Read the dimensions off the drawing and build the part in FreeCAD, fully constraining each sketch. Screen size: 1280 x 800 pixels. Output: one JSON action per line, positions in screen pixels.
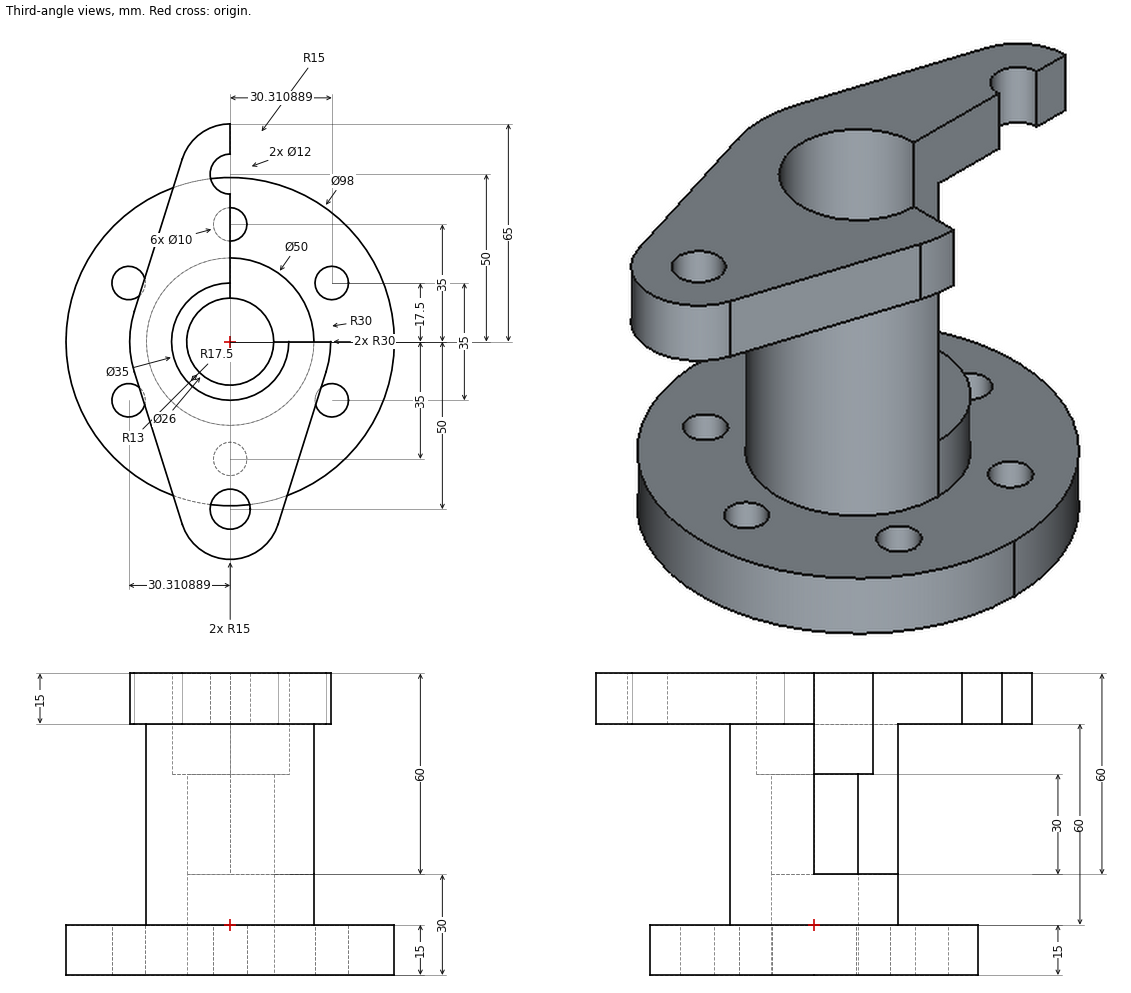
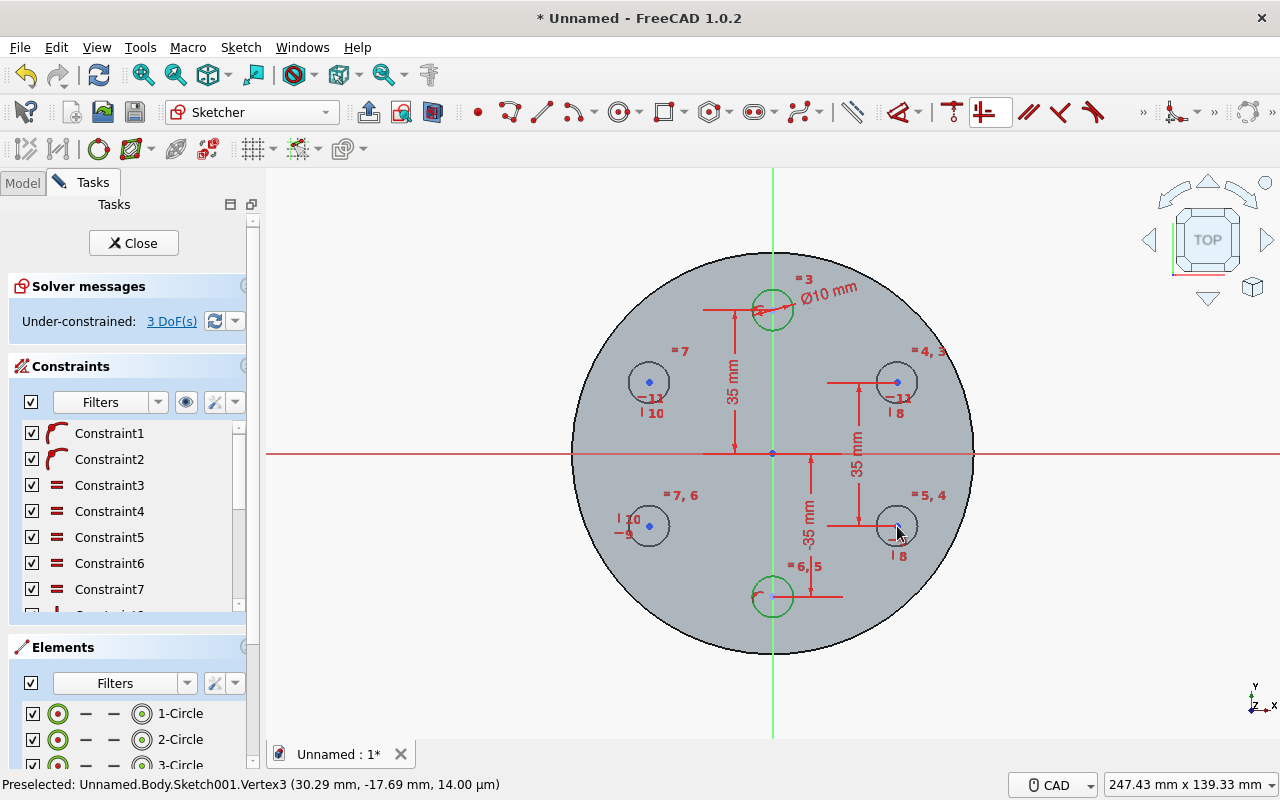
{"action": "left_click", "coordinate": [897, 383]}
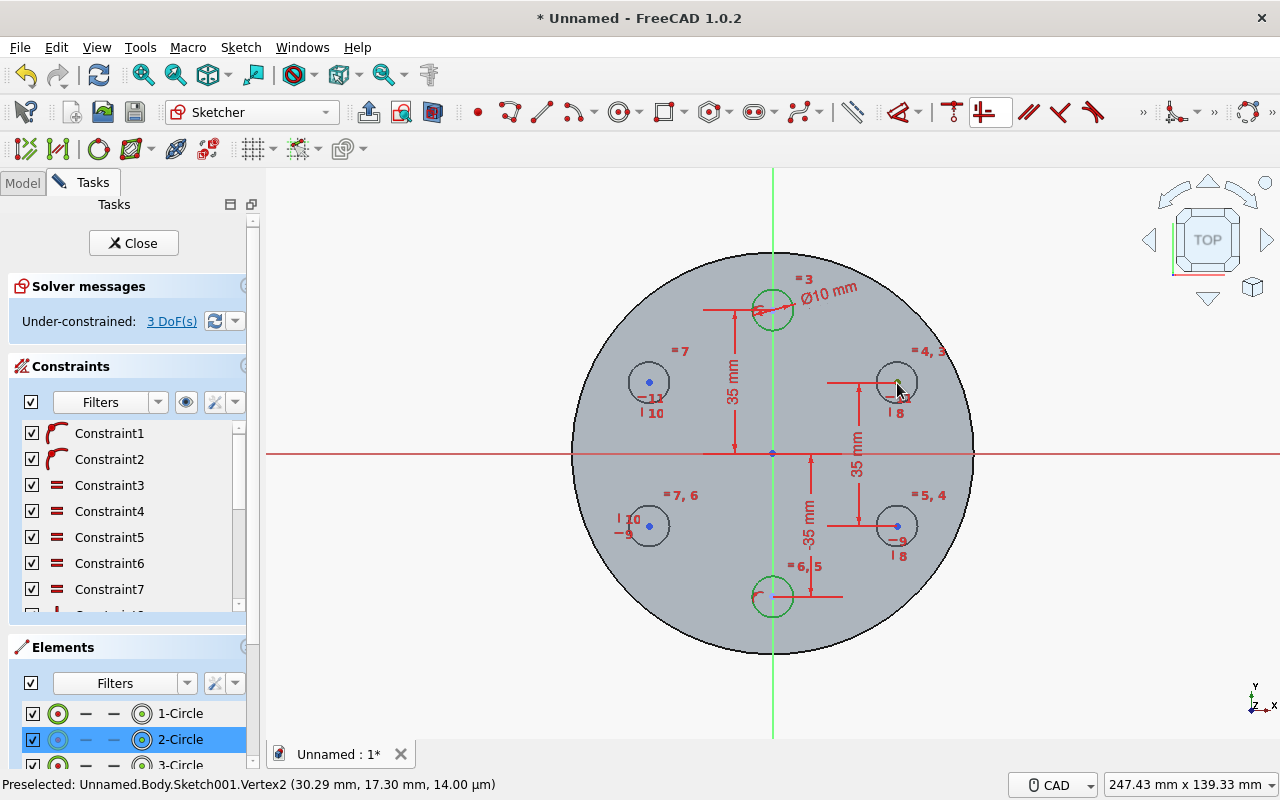
{"action": "key", "text": "i"}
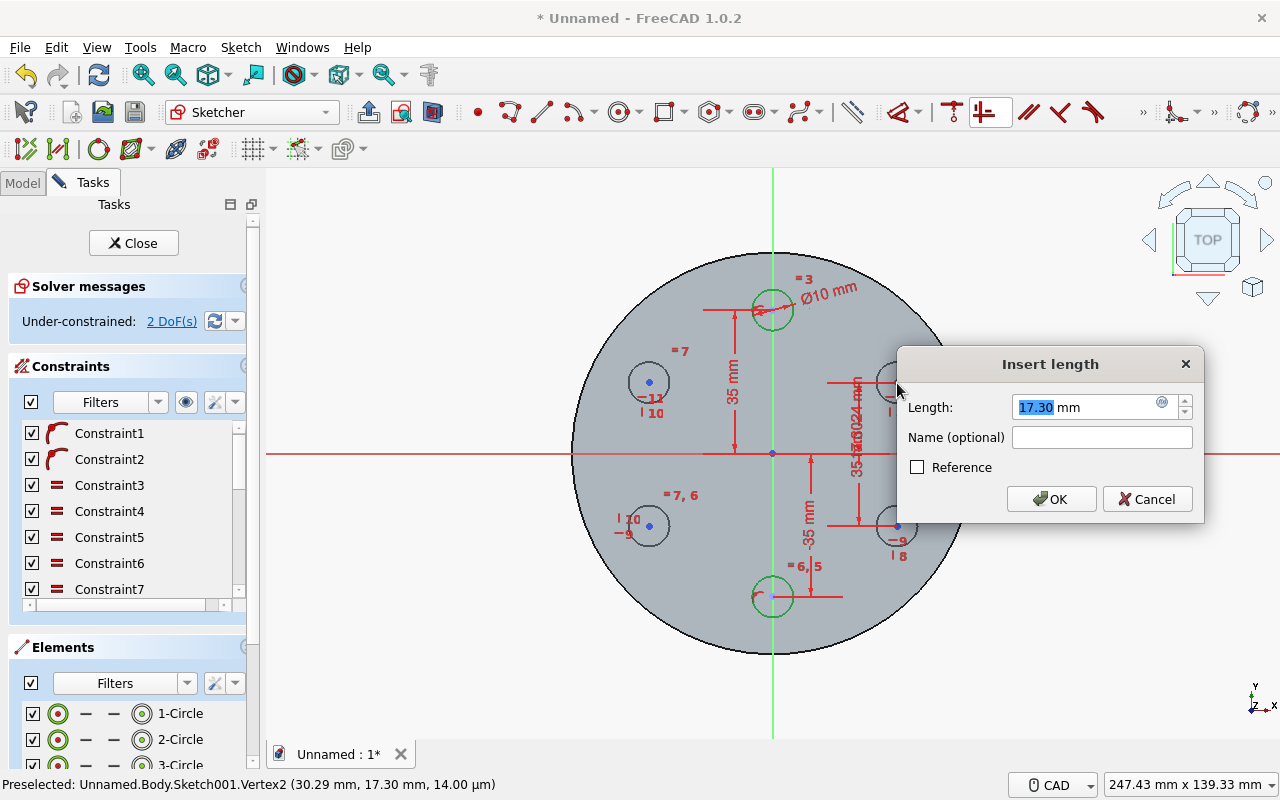
{"action": "type", "text": "17.5"}
{"action": "key", "text": "Return"}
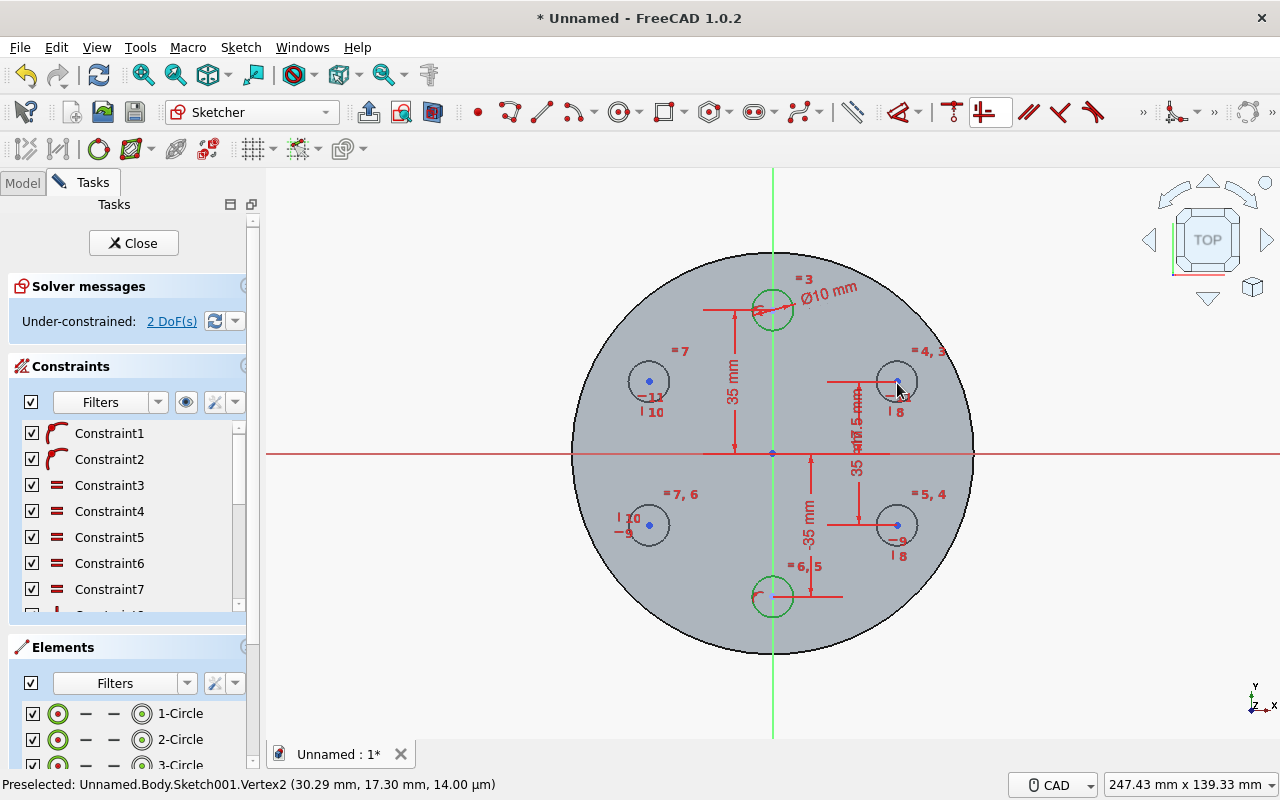
{"action": "left_click", "coordinate": [897, 382]}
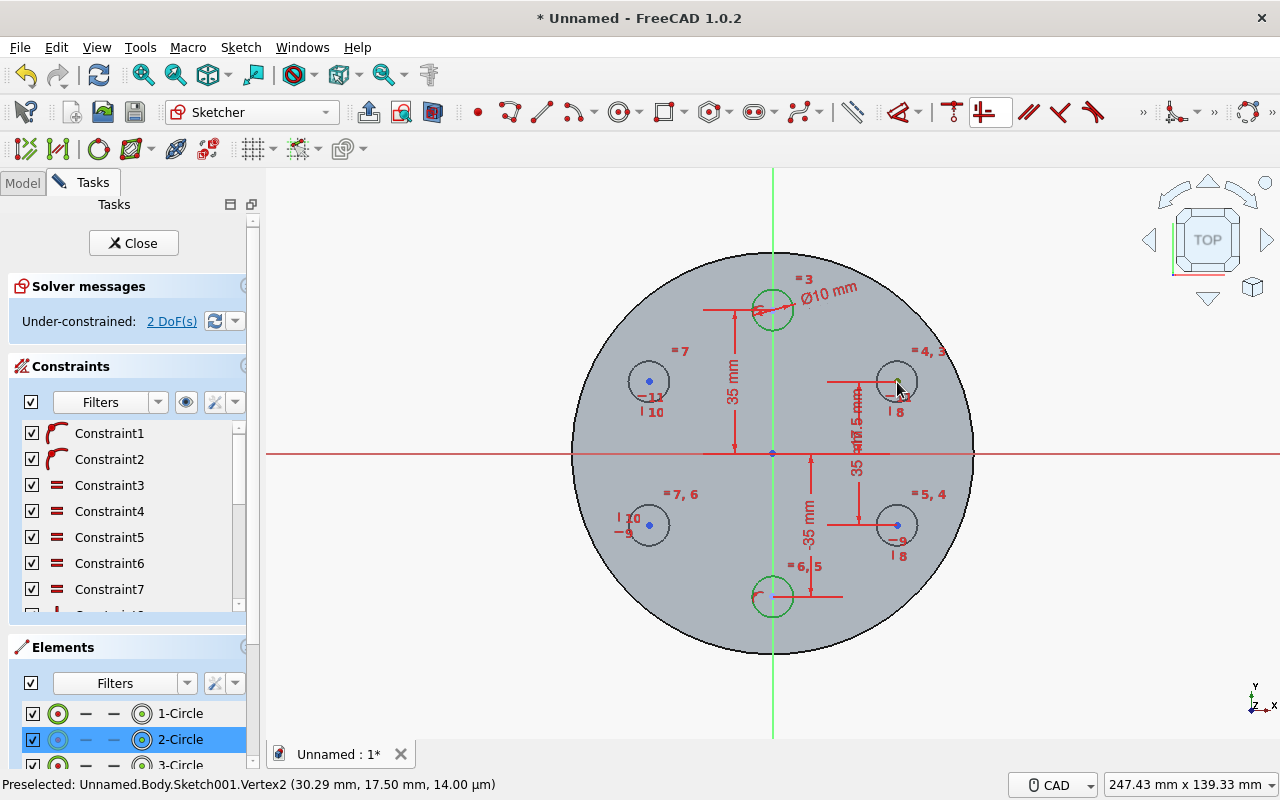
{"action": "key", "text": "l"}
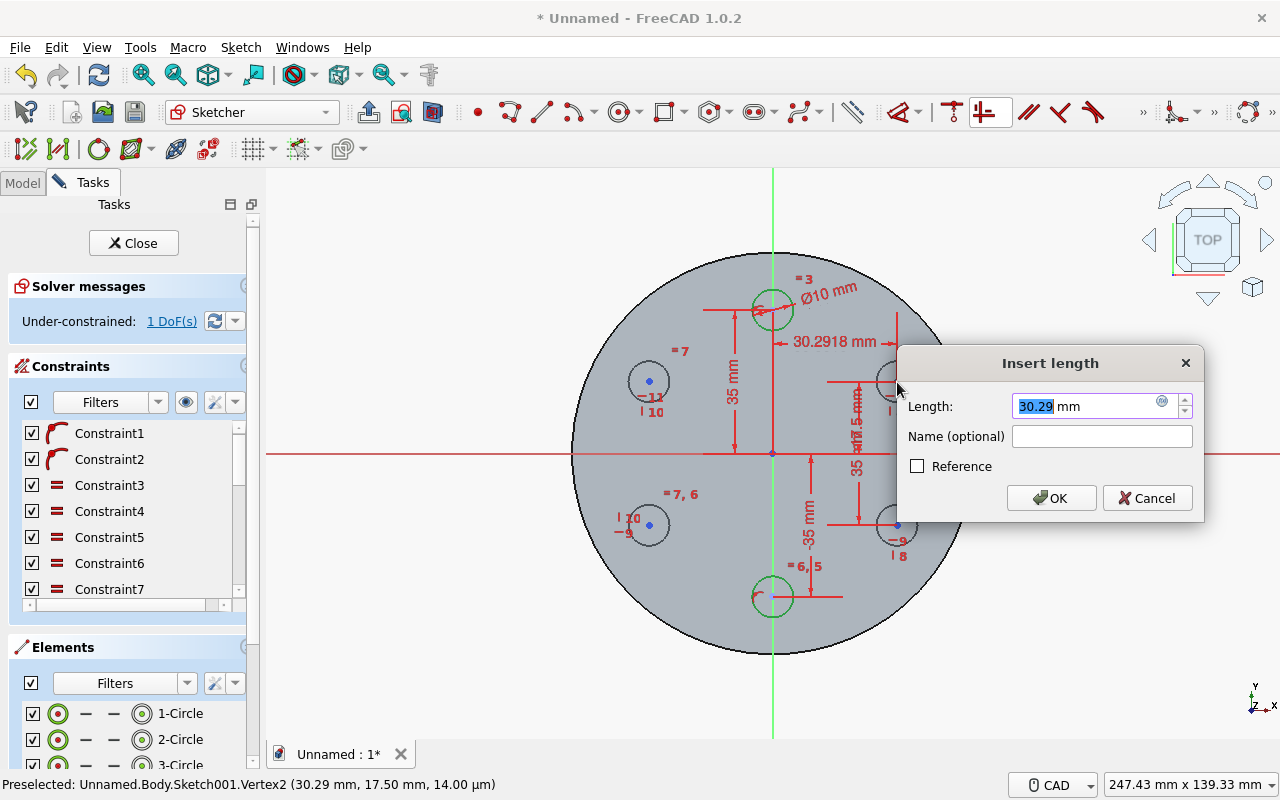
{"action": "type", "text": "30.310889"}
{"action": "key", "text": "Return"}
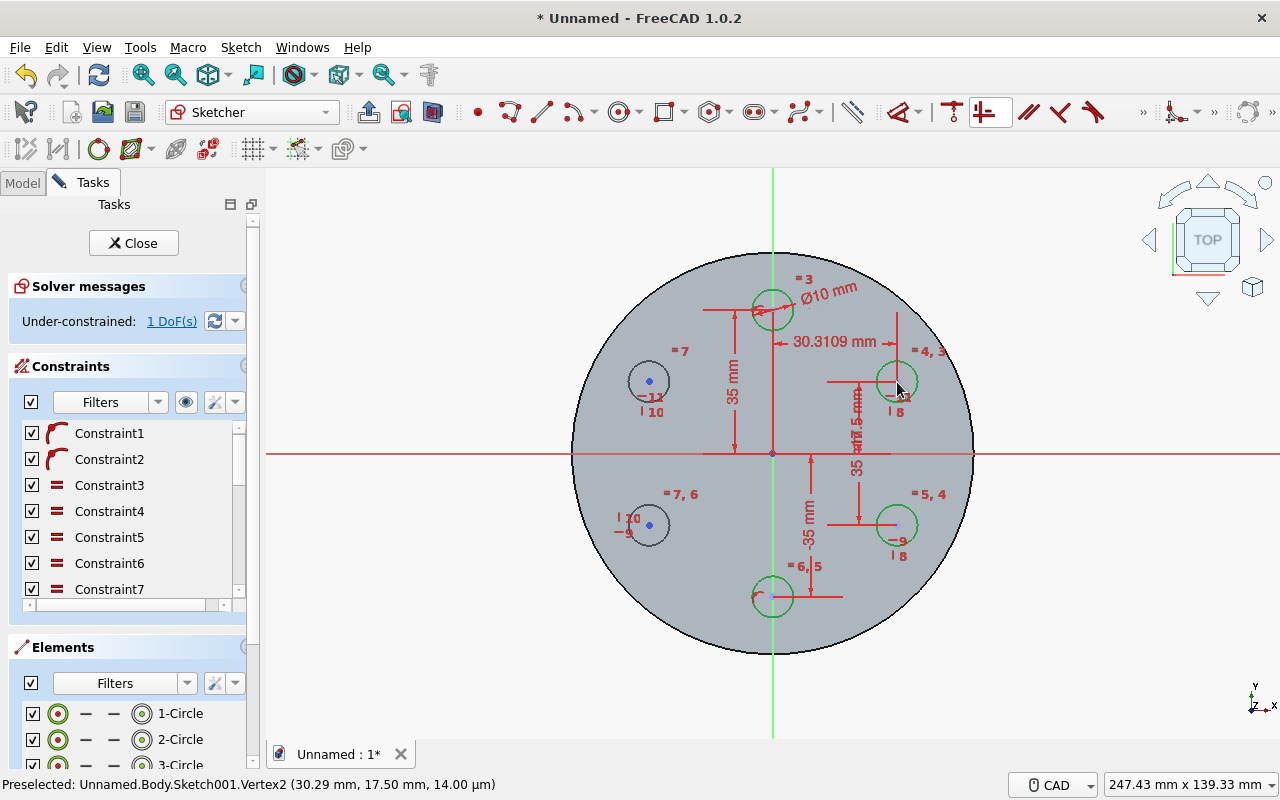
{"action": "left_click", "coordinate": [649, 525]}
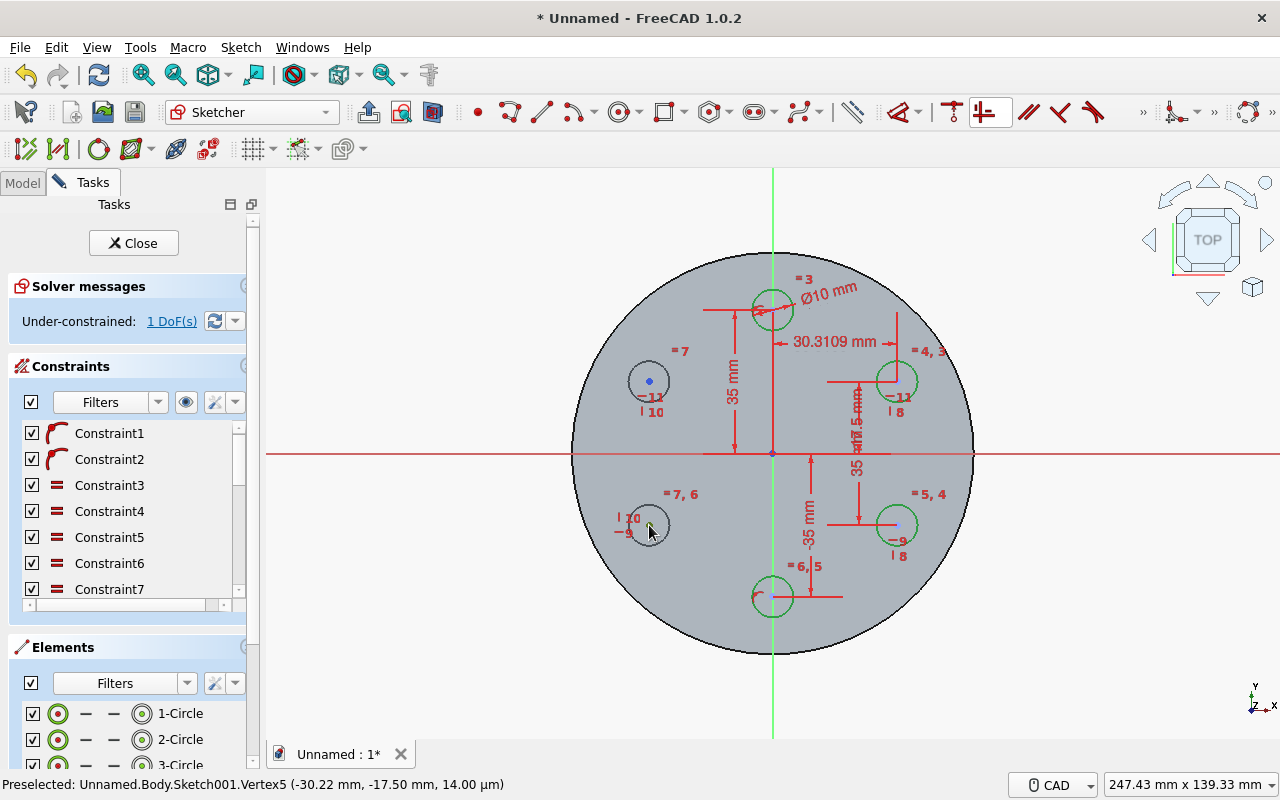
{"action": "key", "text": "l"}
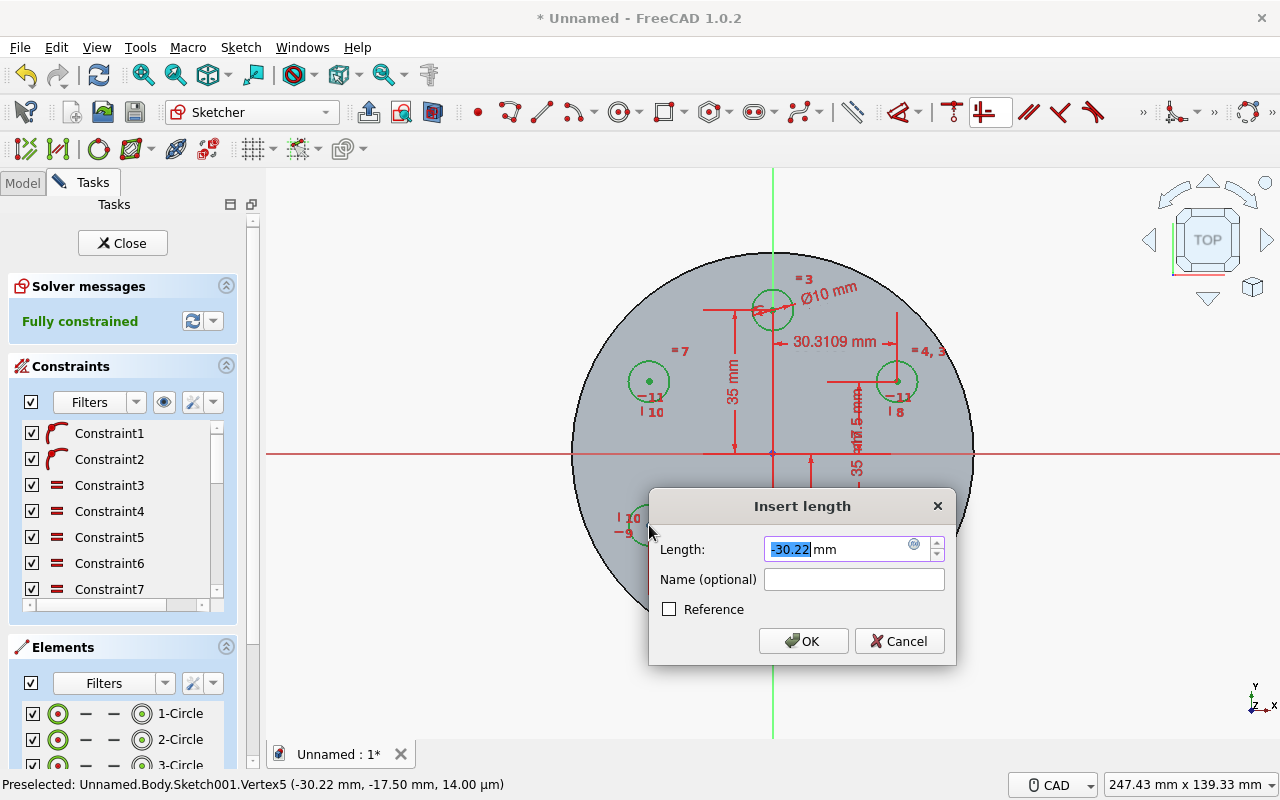
{"action": "type", "text": "-30.310889"}
{"action": "key", "text": "Return"}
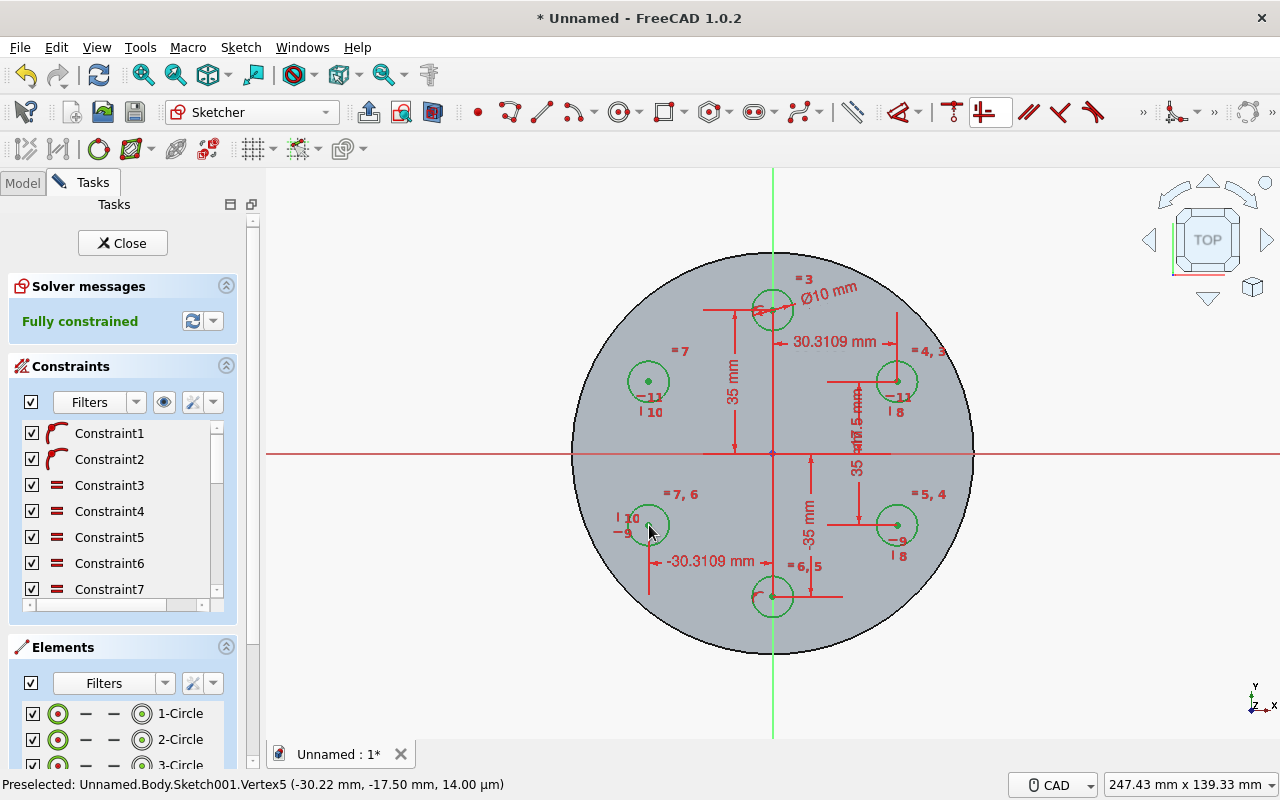
{"action": "left_click", "coordinate": [123, 243]}